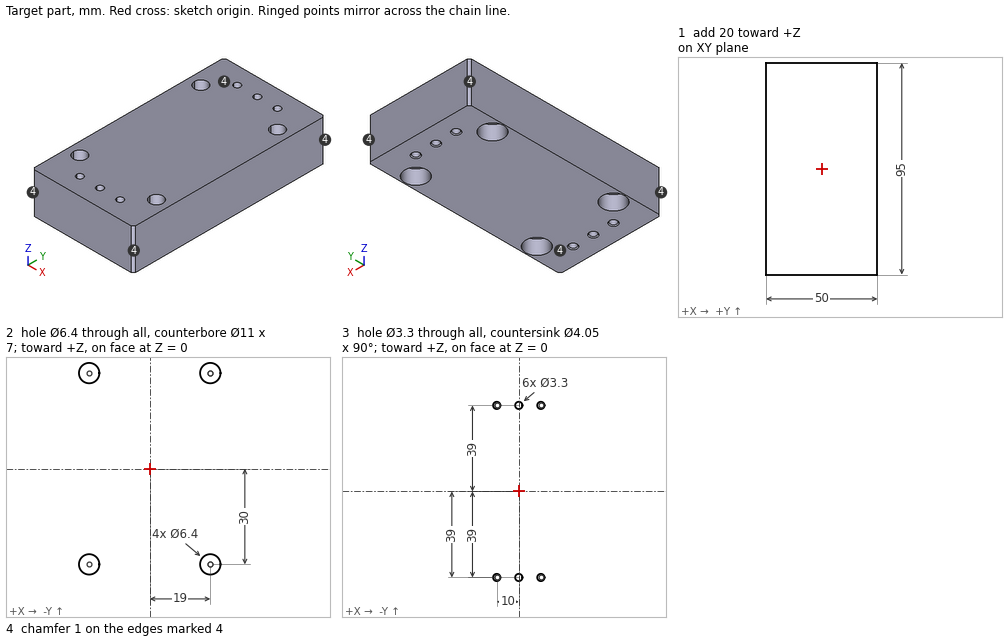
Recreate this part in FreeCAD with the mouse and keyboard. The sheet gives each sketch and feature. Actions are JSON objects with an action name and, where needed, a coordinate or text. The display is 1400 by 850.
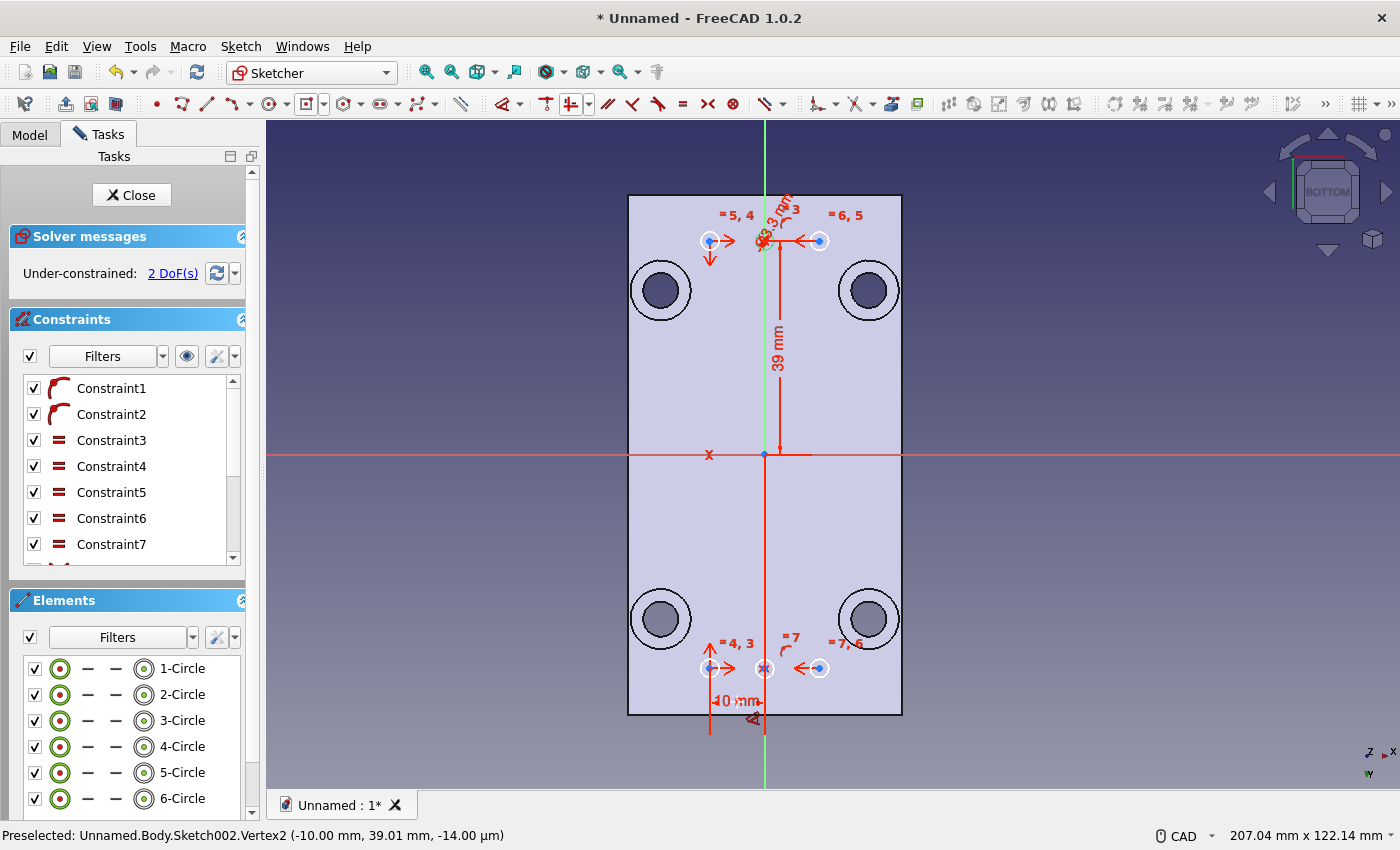
{"action": "left_click", "coordinate": [710, 668]}
{"action": "left_click", "coordinate": [676, 562]}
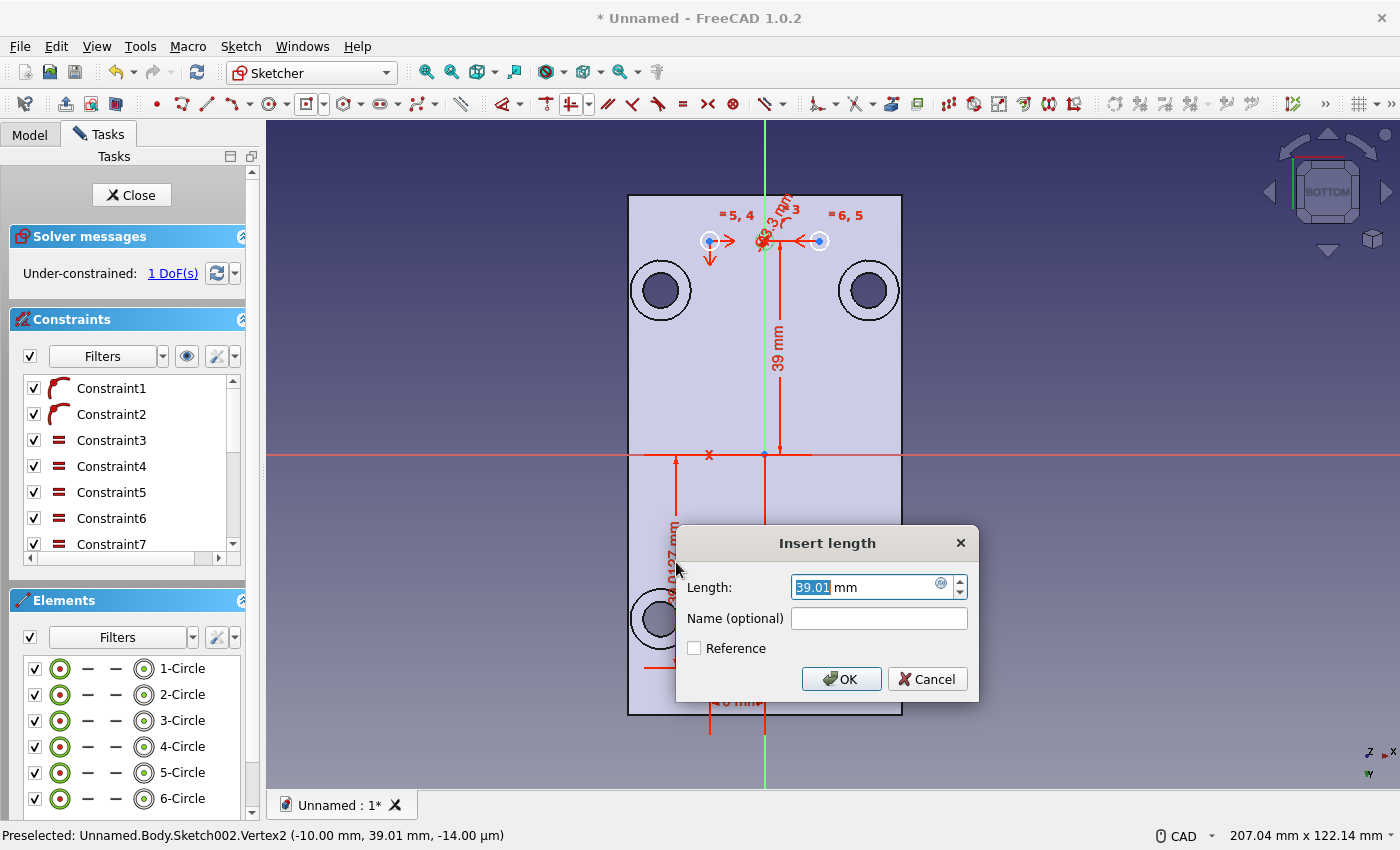
{"action": "type", "text": "39"}
{"action": "key", "text": "Return"}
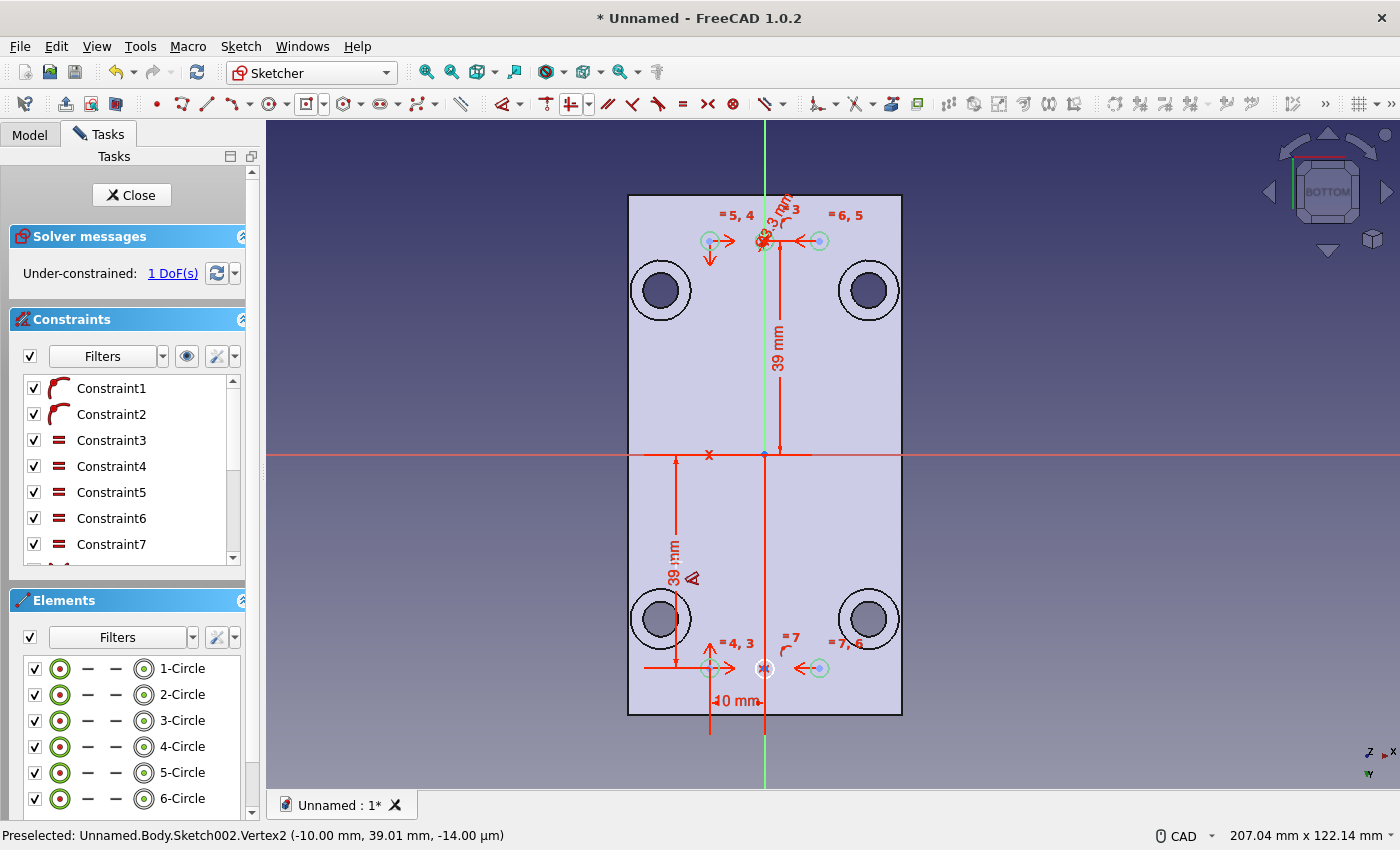
{"action": "left_click", "coordinate": [765, 669]}
{"action": "left_click", "coordinate": [799, 562]}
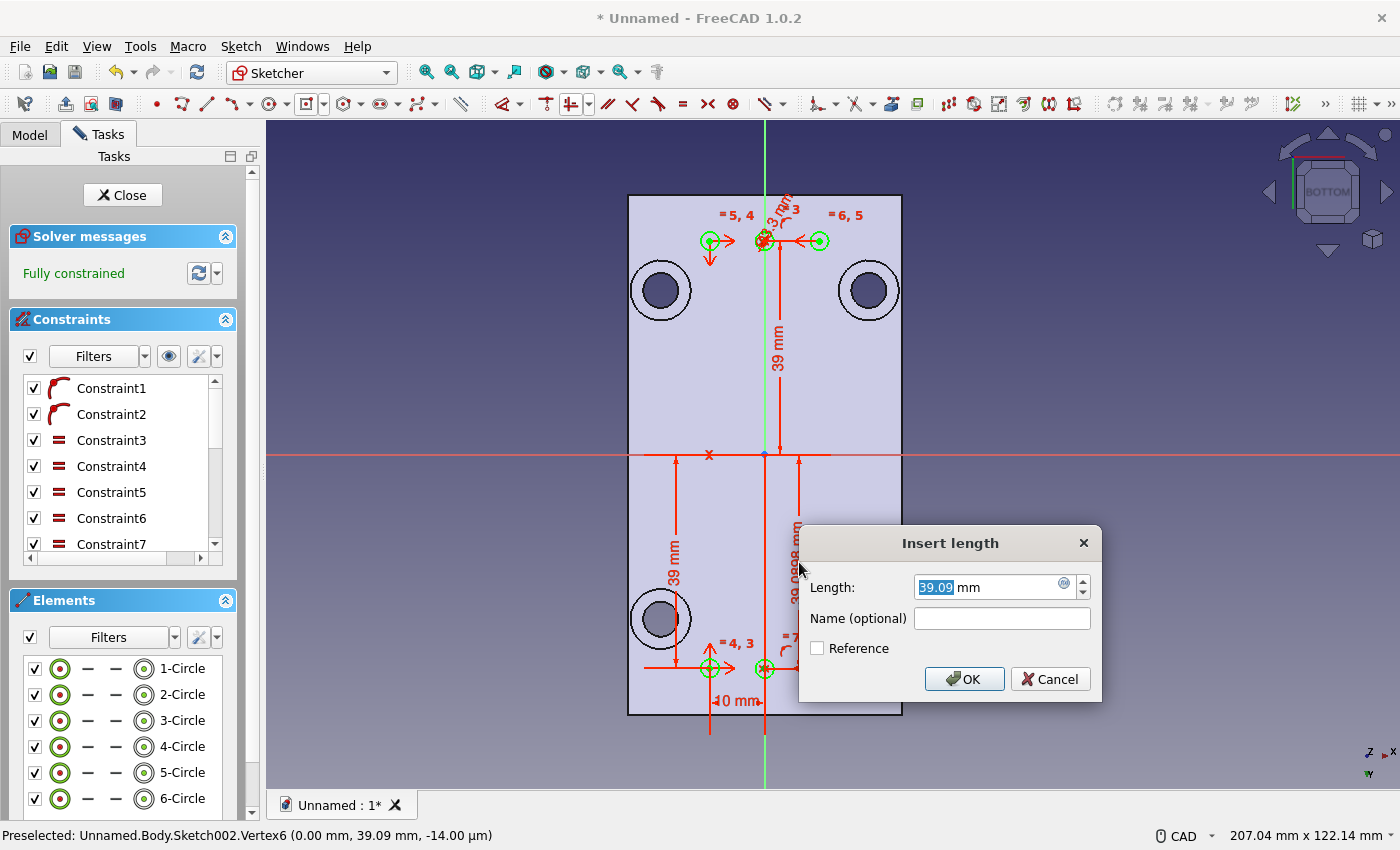
{"action": "type", "text": "39"}
{"action": "key", "text": "Return"}
{"action": "key", "text": "Escape"}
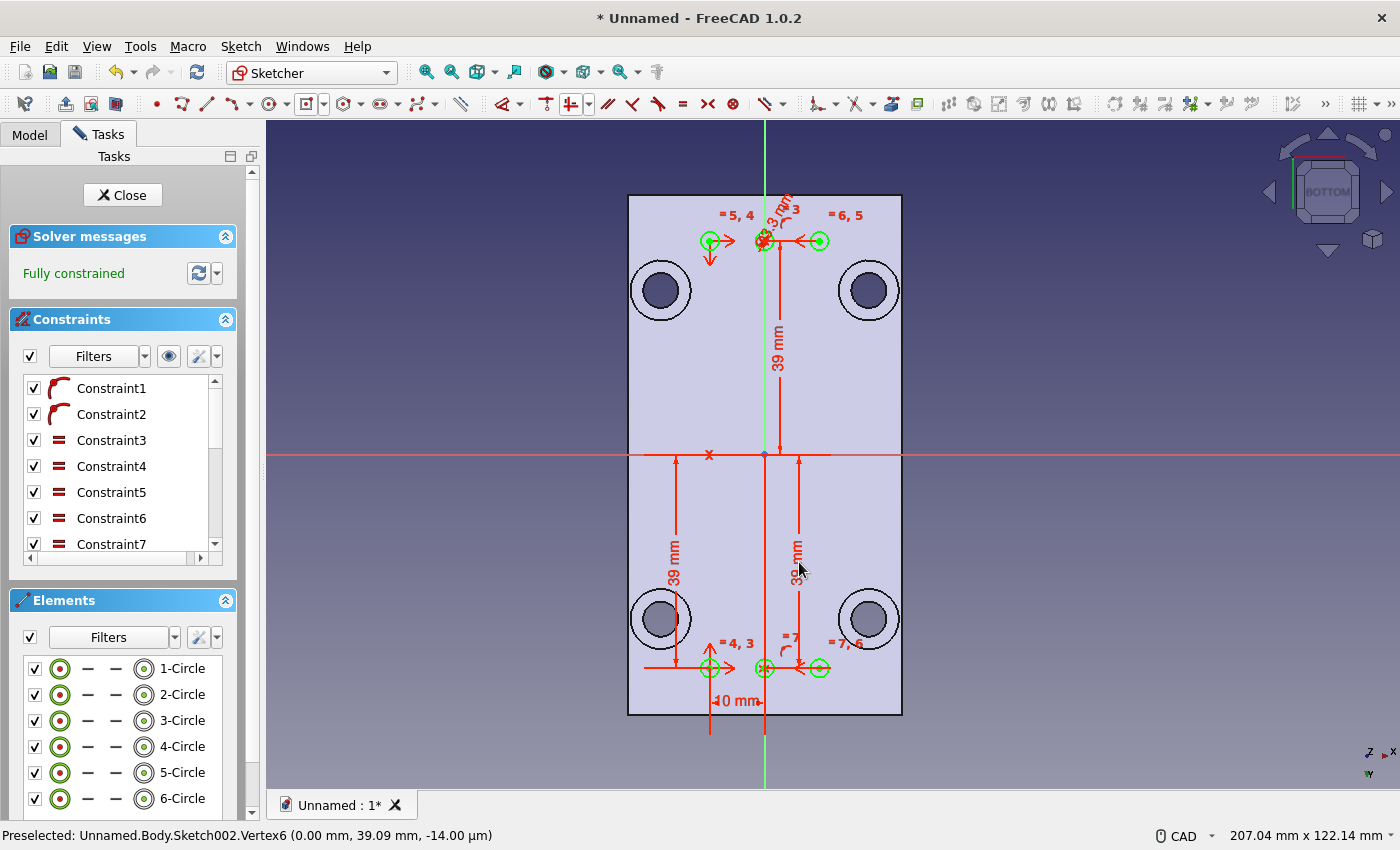
{"action": "left_click", "coordinate": [123, 195]}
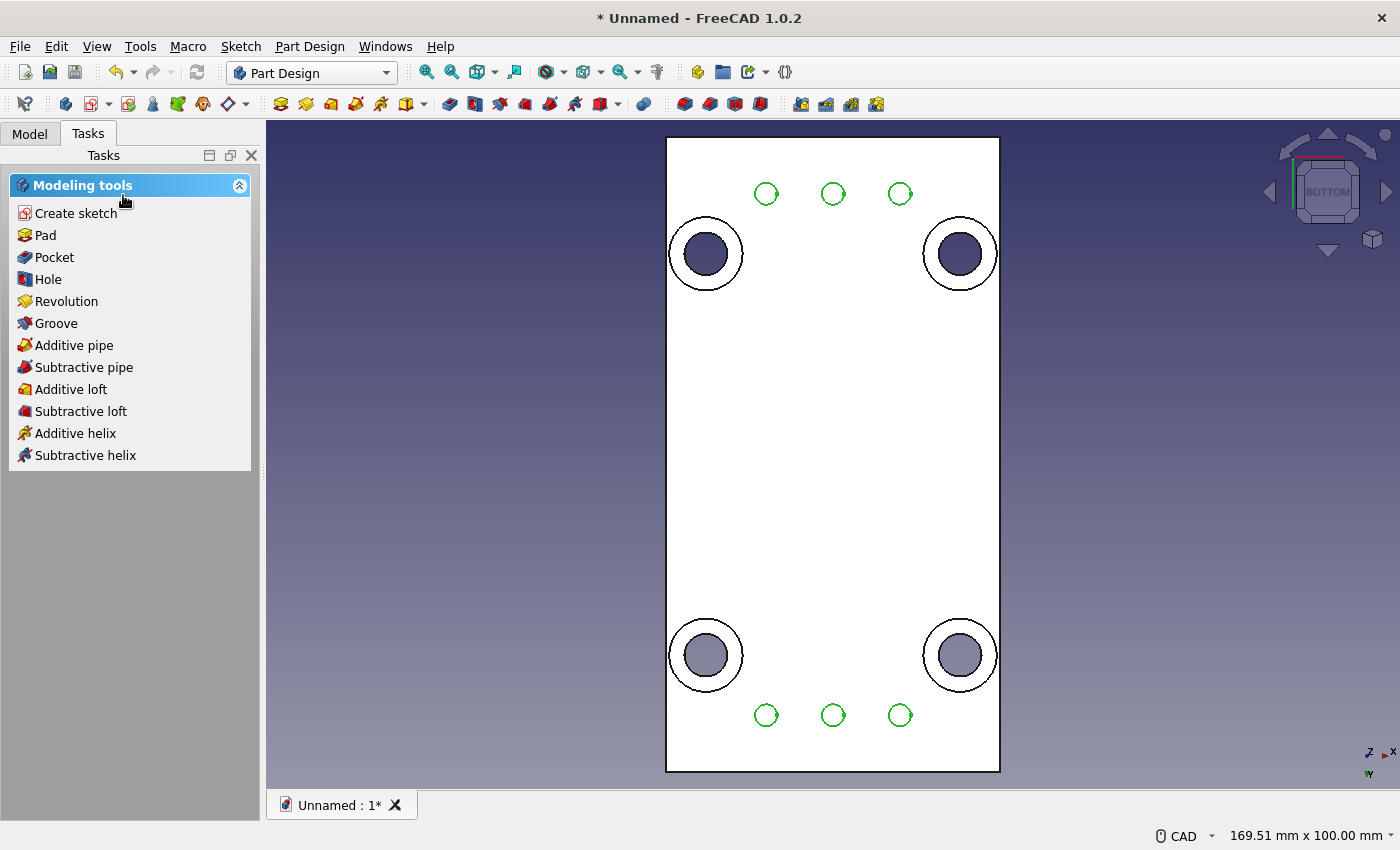
{"action": "left_click", "coordinate": [475, 104]}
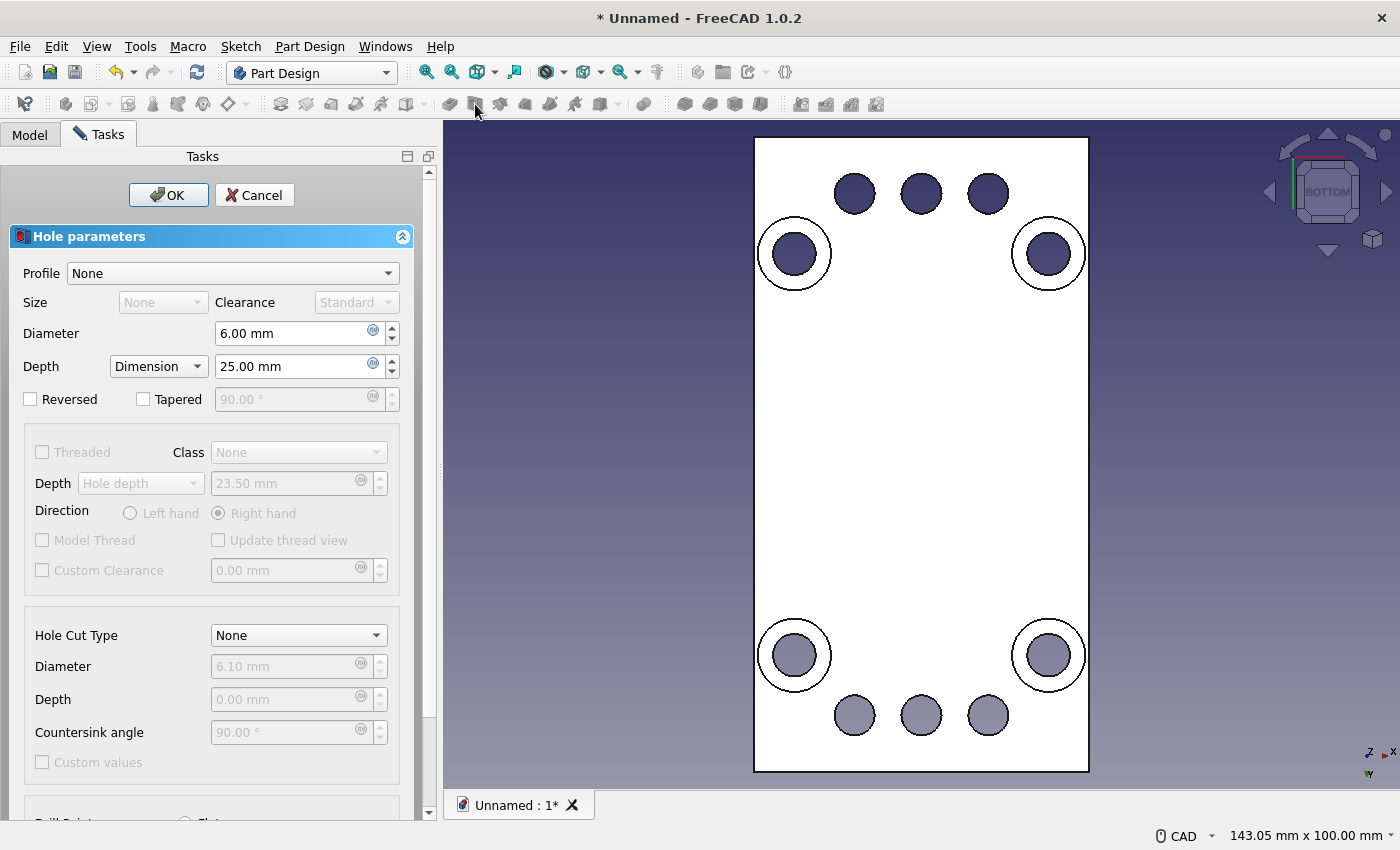
{"action": "triple_click", "coordinate": [300, 334]}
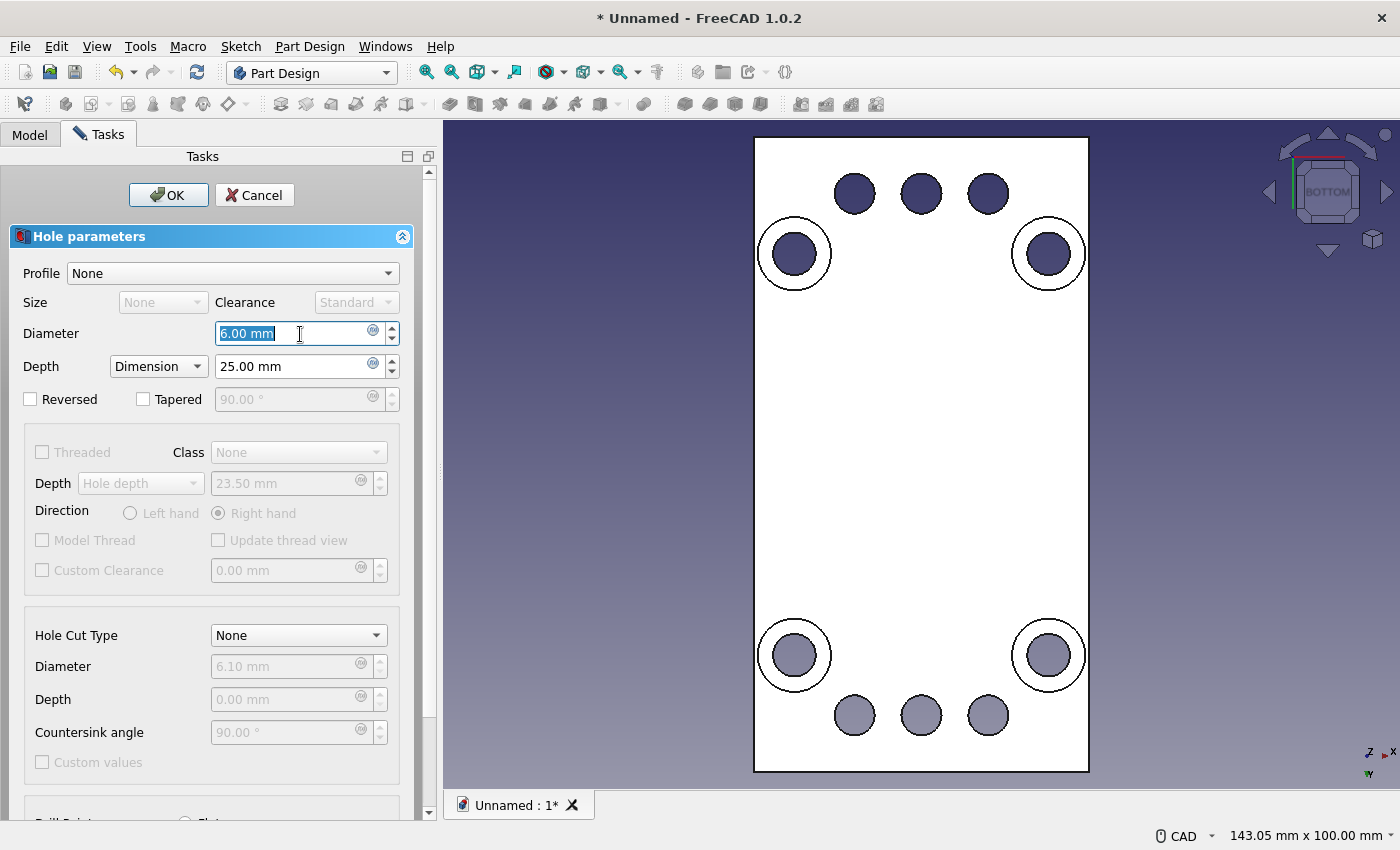
{"action": "type", "text": "3.3"}
{"action": "key", "text": "Tab"}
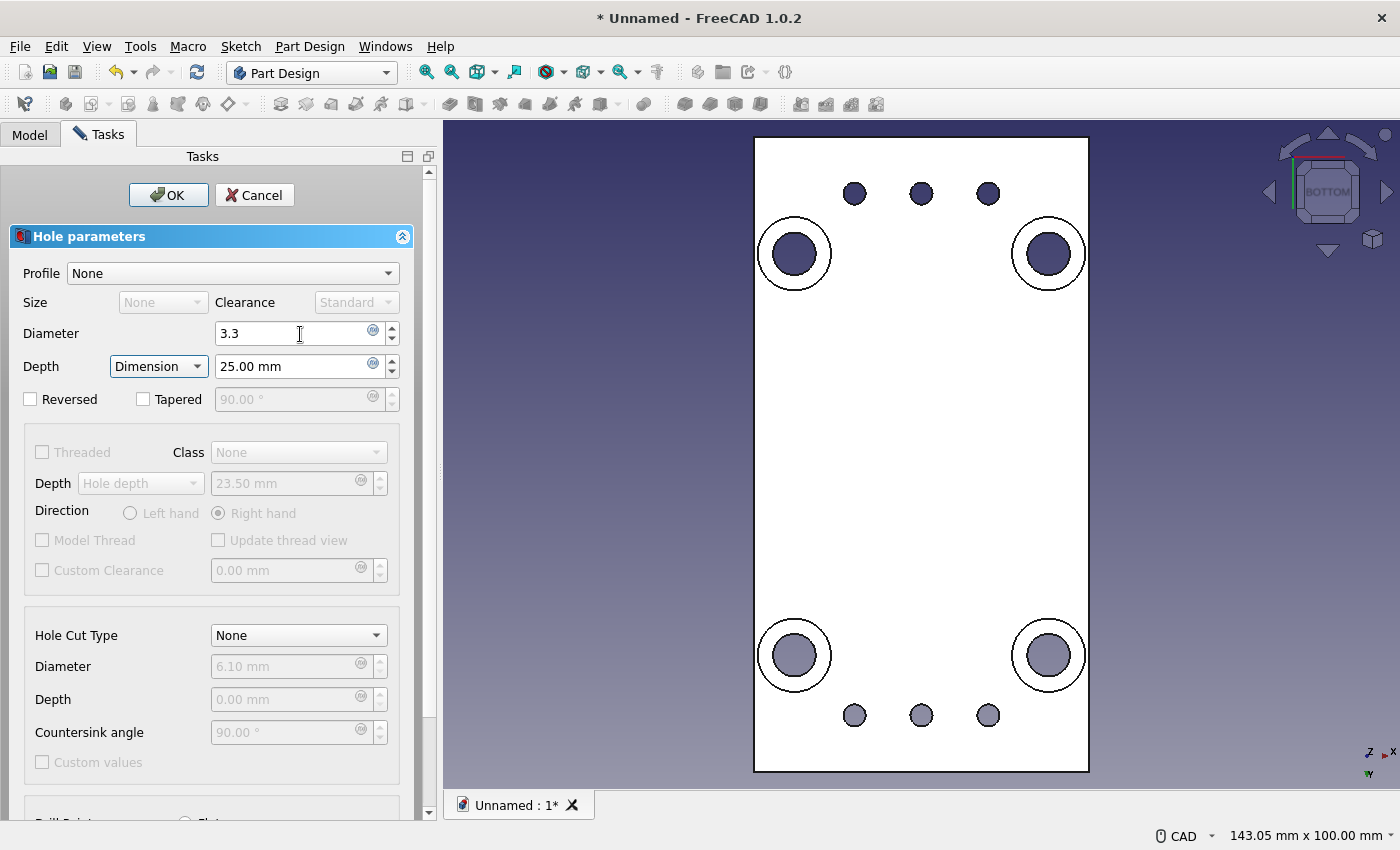
{"action": "left_click", "coordinate": [160, 366]}